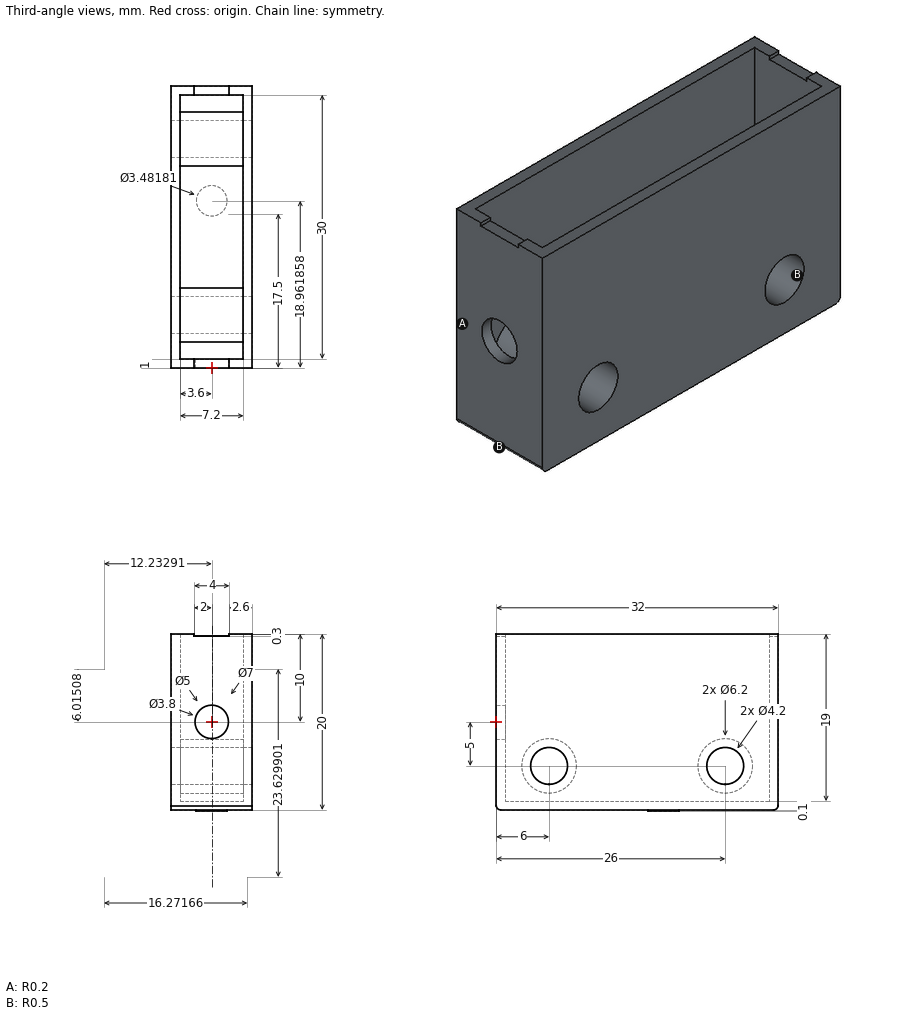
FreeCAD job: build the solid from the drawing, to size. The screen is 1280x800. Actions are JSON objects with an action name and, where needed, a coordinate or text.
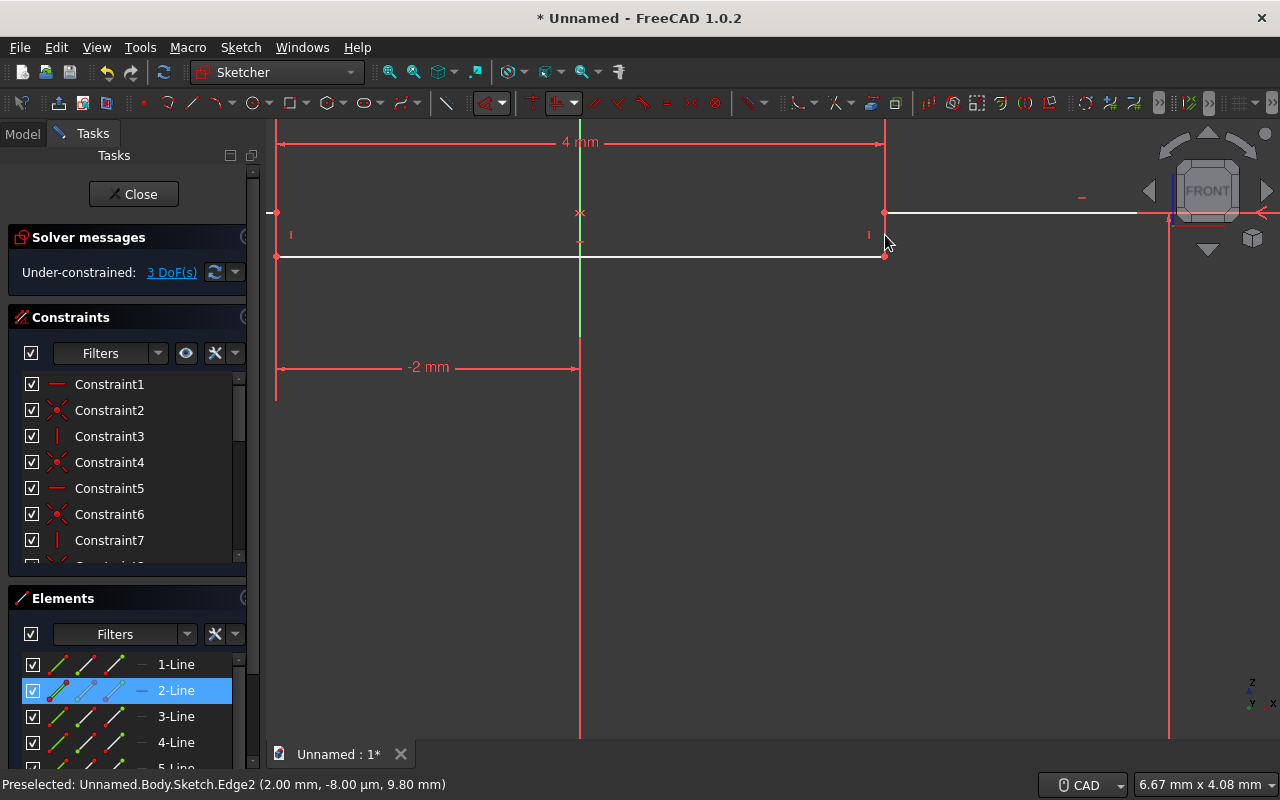
{"action": "left_click", "coordinate": [504, 104]}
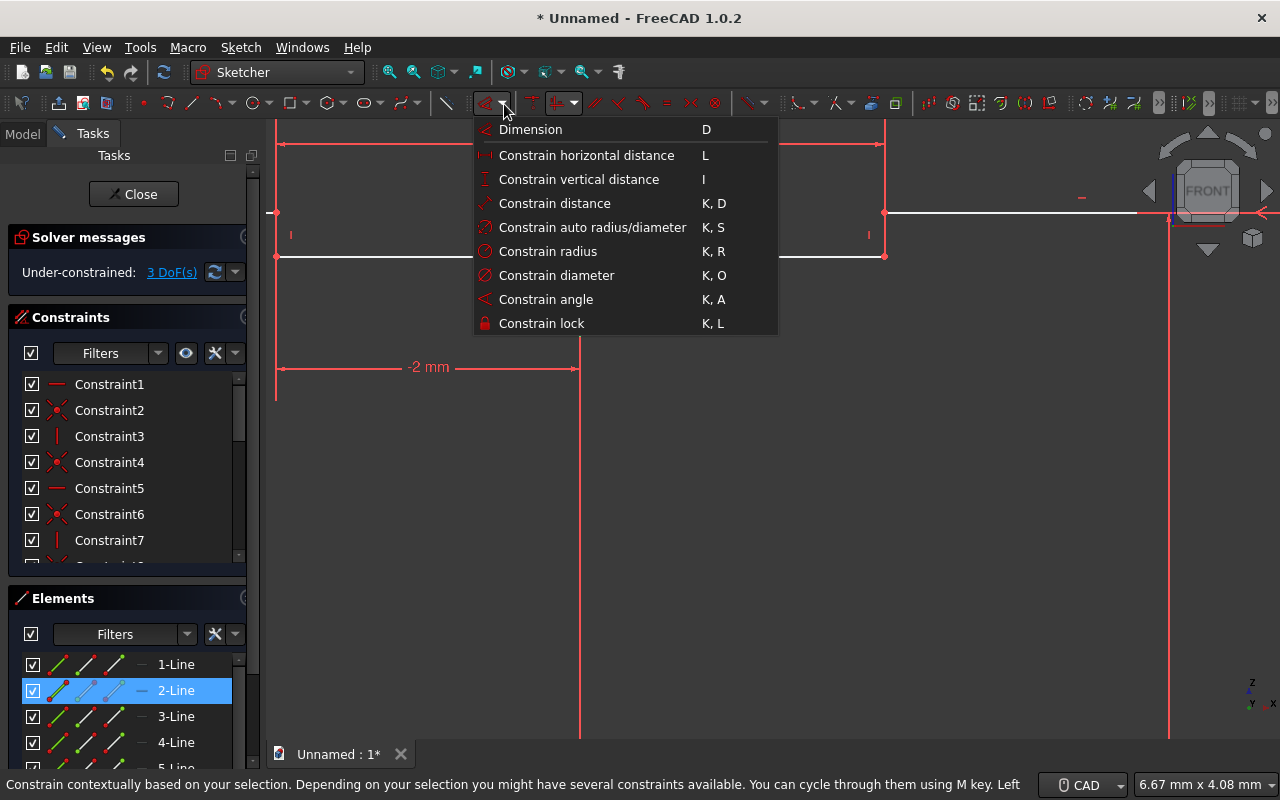
{"action": "left_click", "coordinate": [626, 179]}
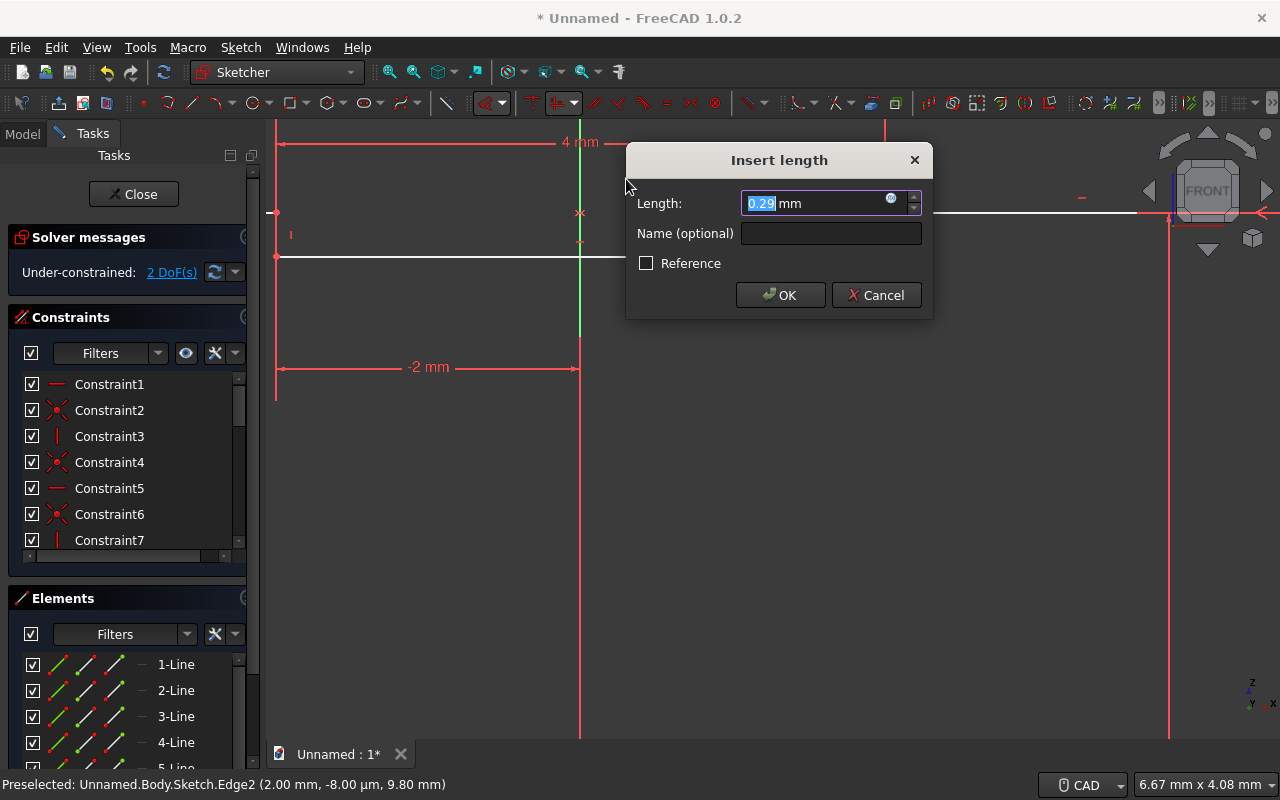
{"action": "type", "text": "0.3"}
{"action": "key", "text": "Return"}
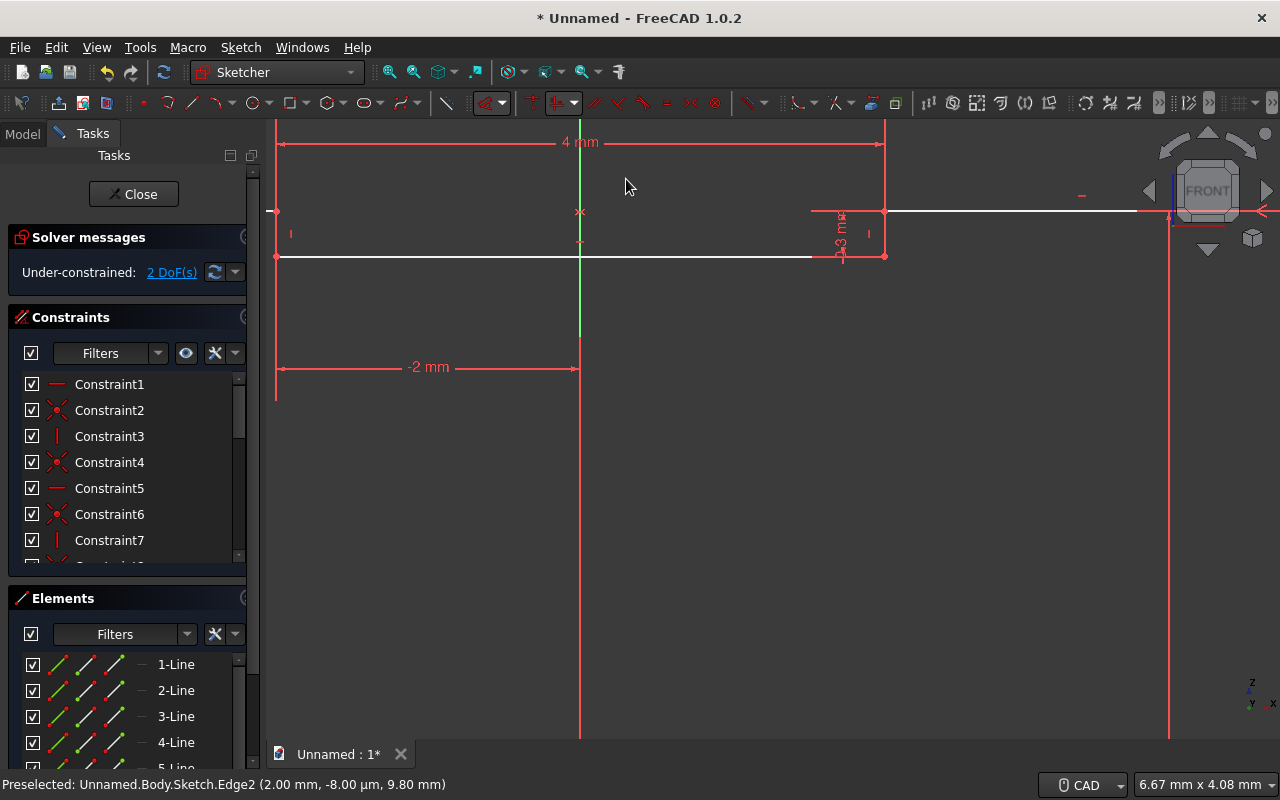
{"action": "scroll", "coordinate": [724, 226], "scroll_direction": "down", "scroll_amount": 10}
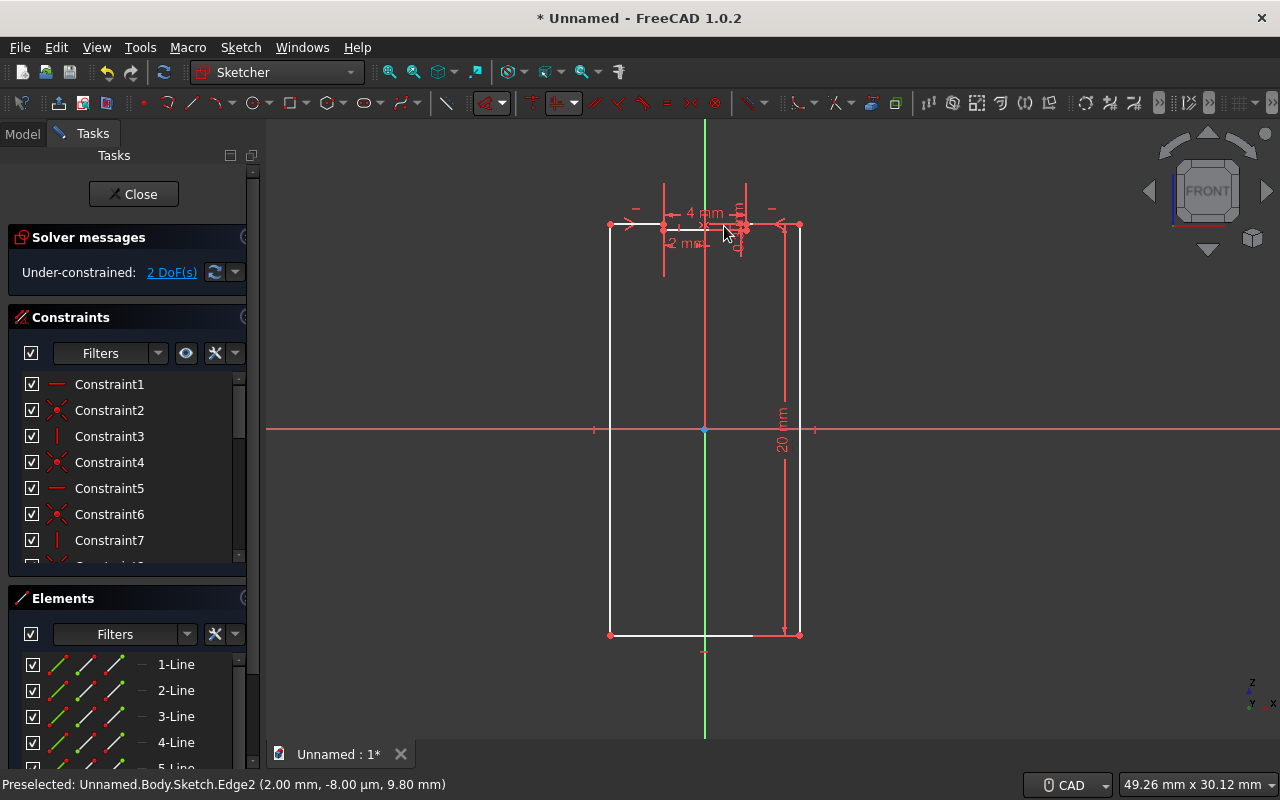
{"action": "left_click", "coordinate": [762, 224]}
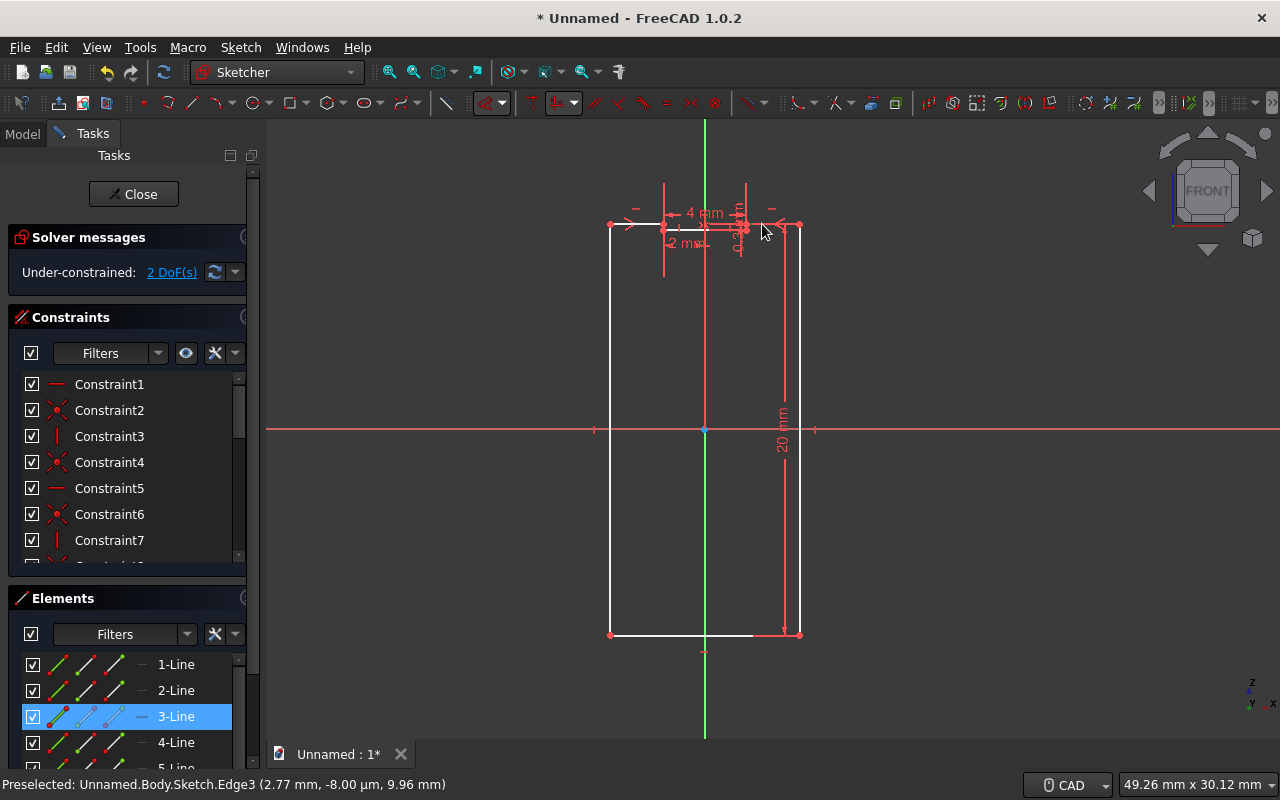
{"action": "left_click", "coordinate": [504, 104]}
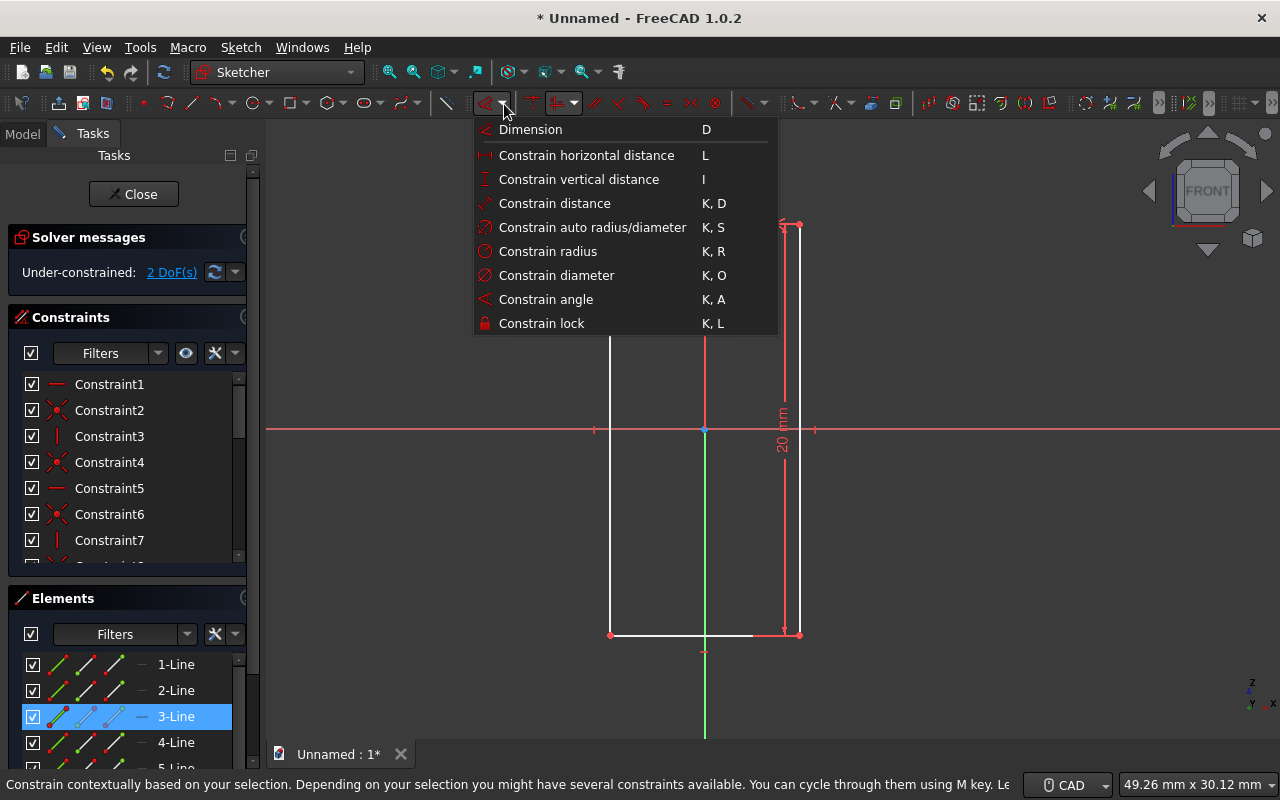
{"action": "left_click", "coordinate": [626, 155]}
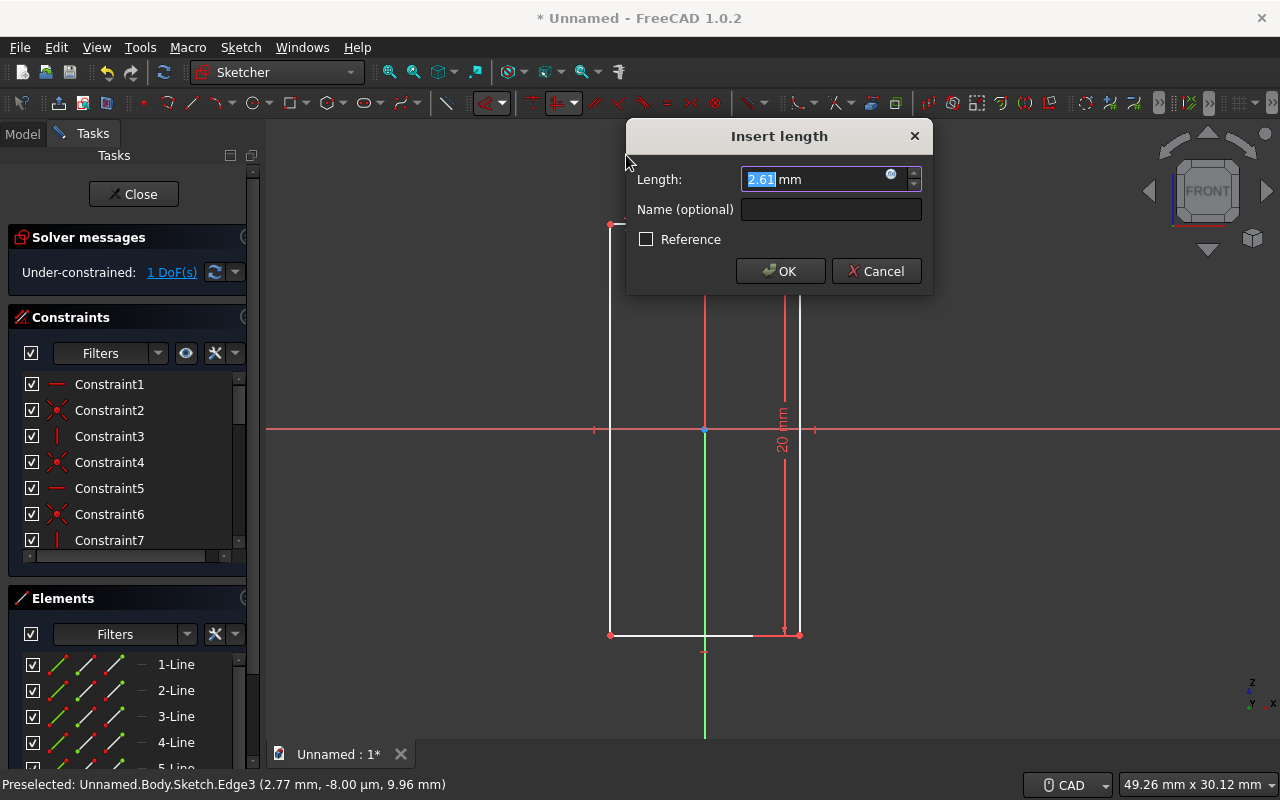
{"action": "type", "text": "2.6"}
{"action": "key", "text": "Return"}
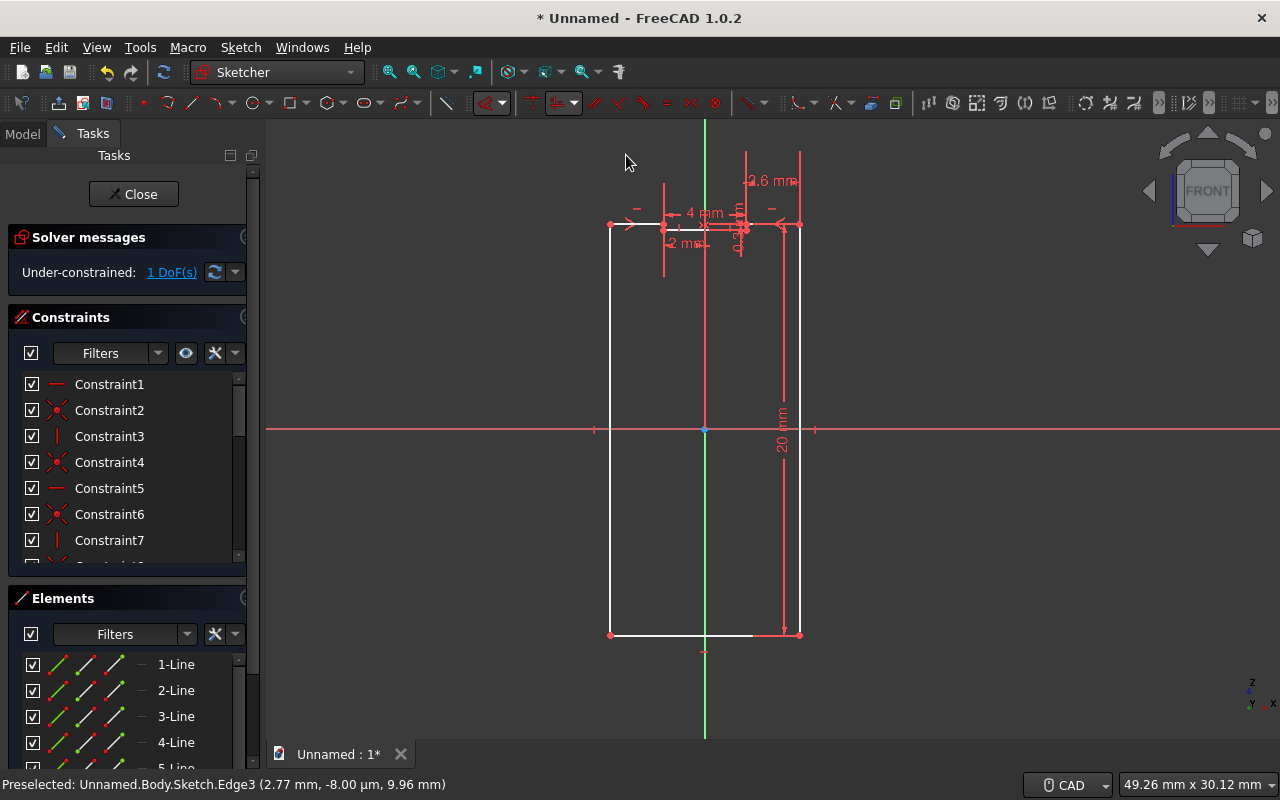
{"action": "scroll", "coordinate": [746, 224], "scroll_direction": "up", "scroll_amount": 4}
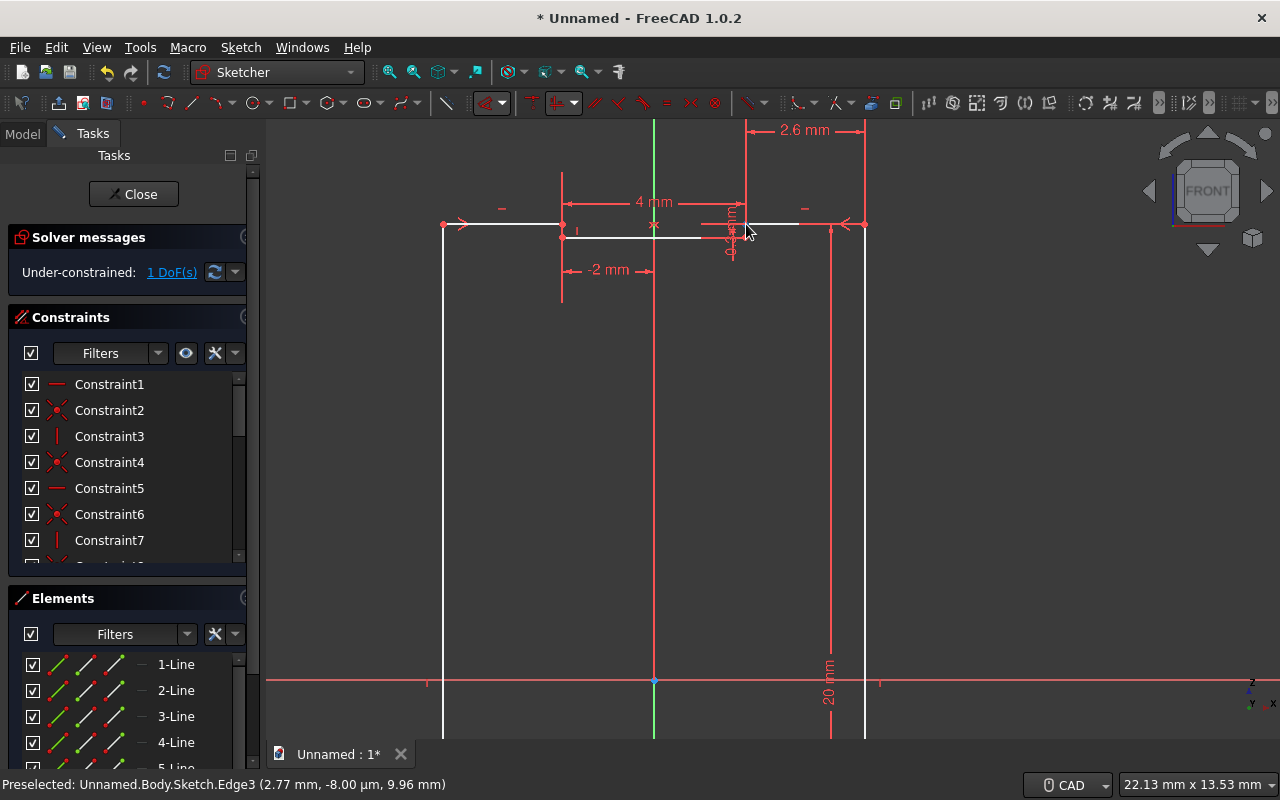
{"action": "left_click", "coordinate": [746, 224]}